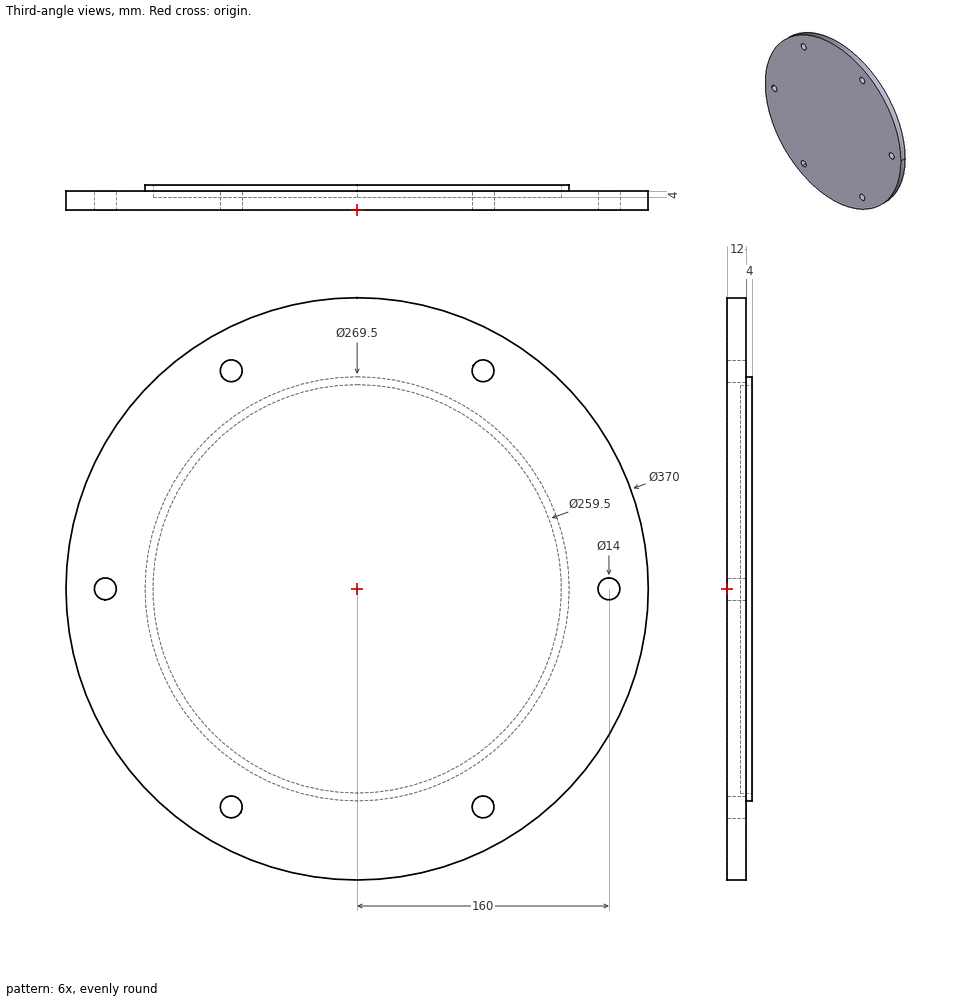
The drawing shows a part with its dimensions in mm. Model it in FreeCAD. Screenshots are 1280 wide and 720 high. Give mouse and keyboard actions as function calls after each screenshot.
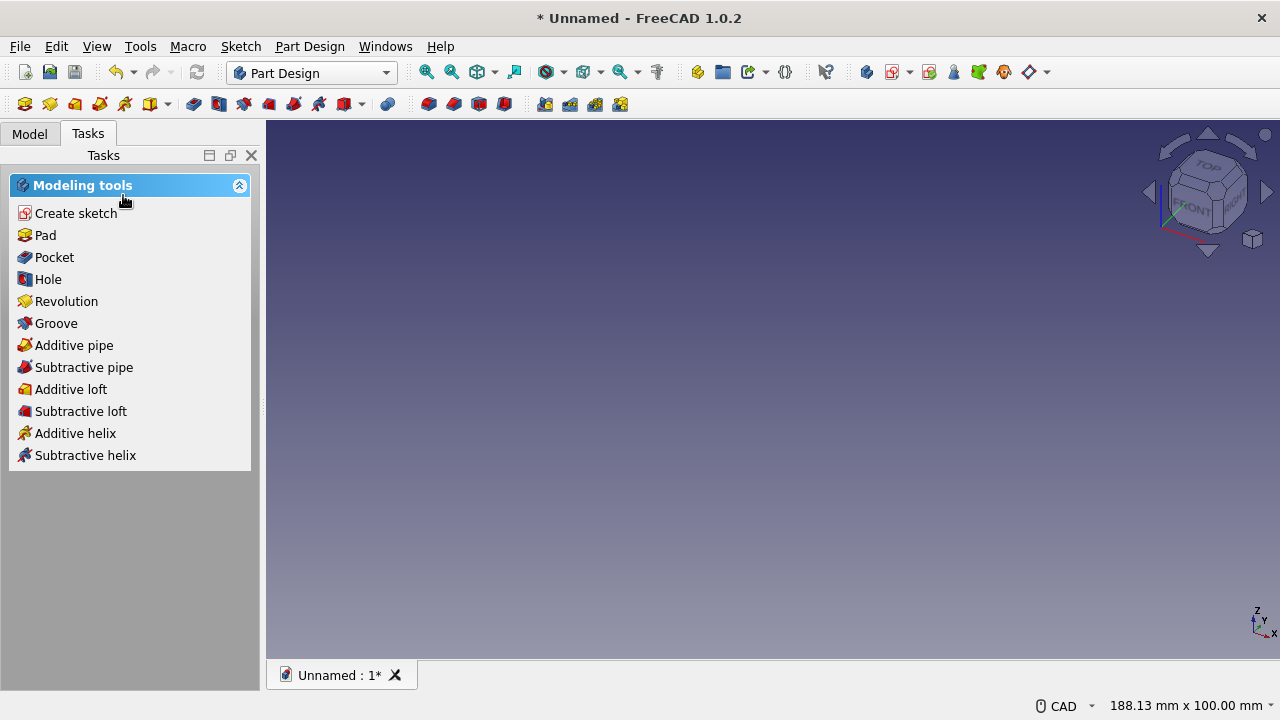
click(25, 104)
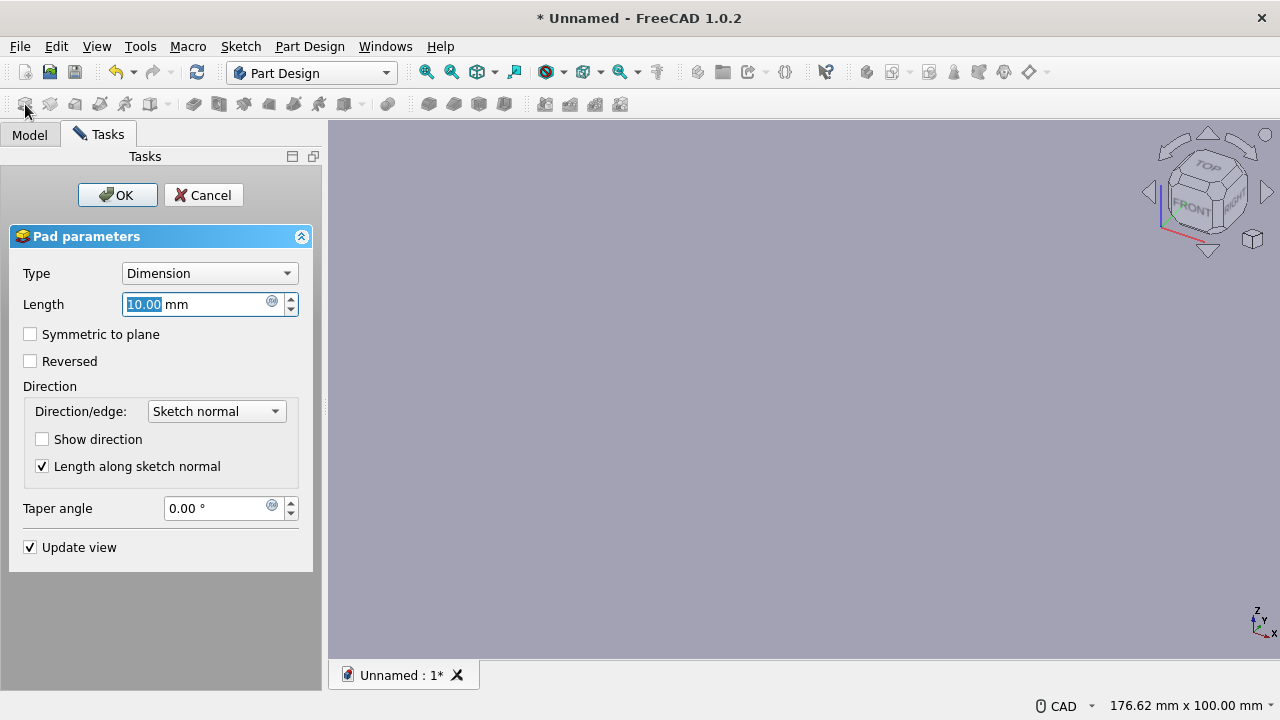
text(12)
key(Tab)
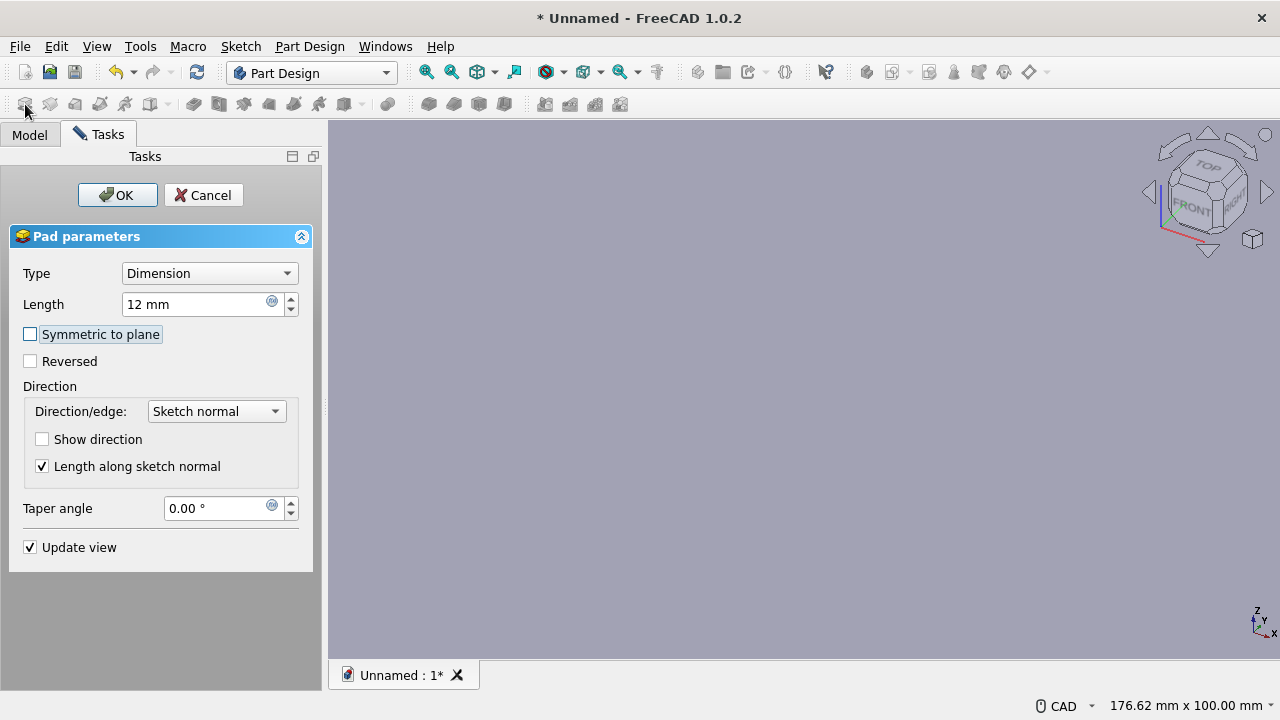
click(31, 361)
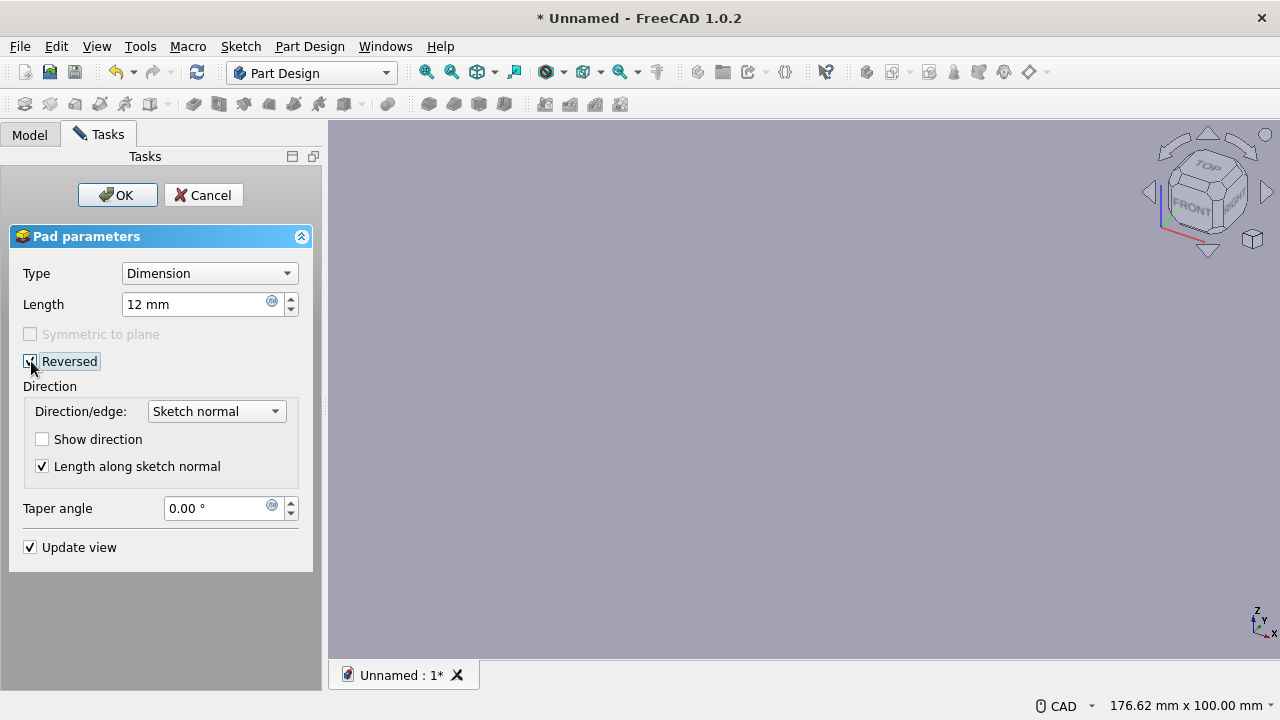
click(118, 195)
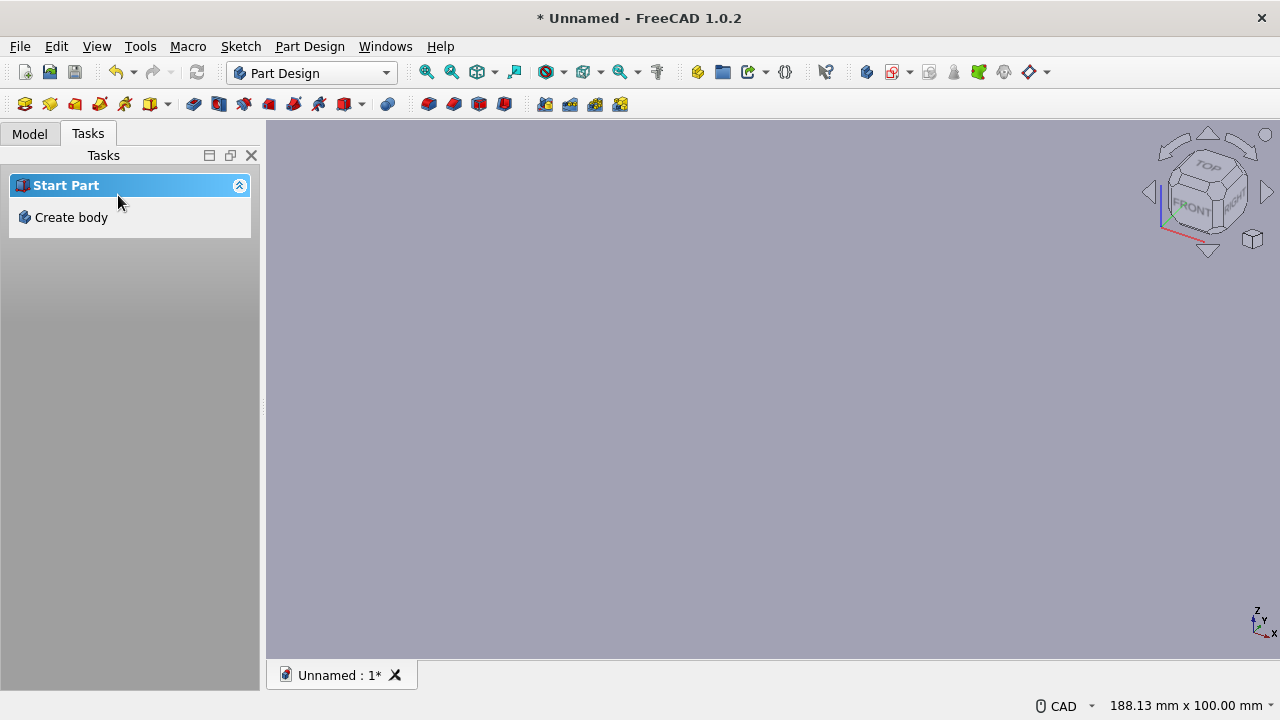
click(427, 72)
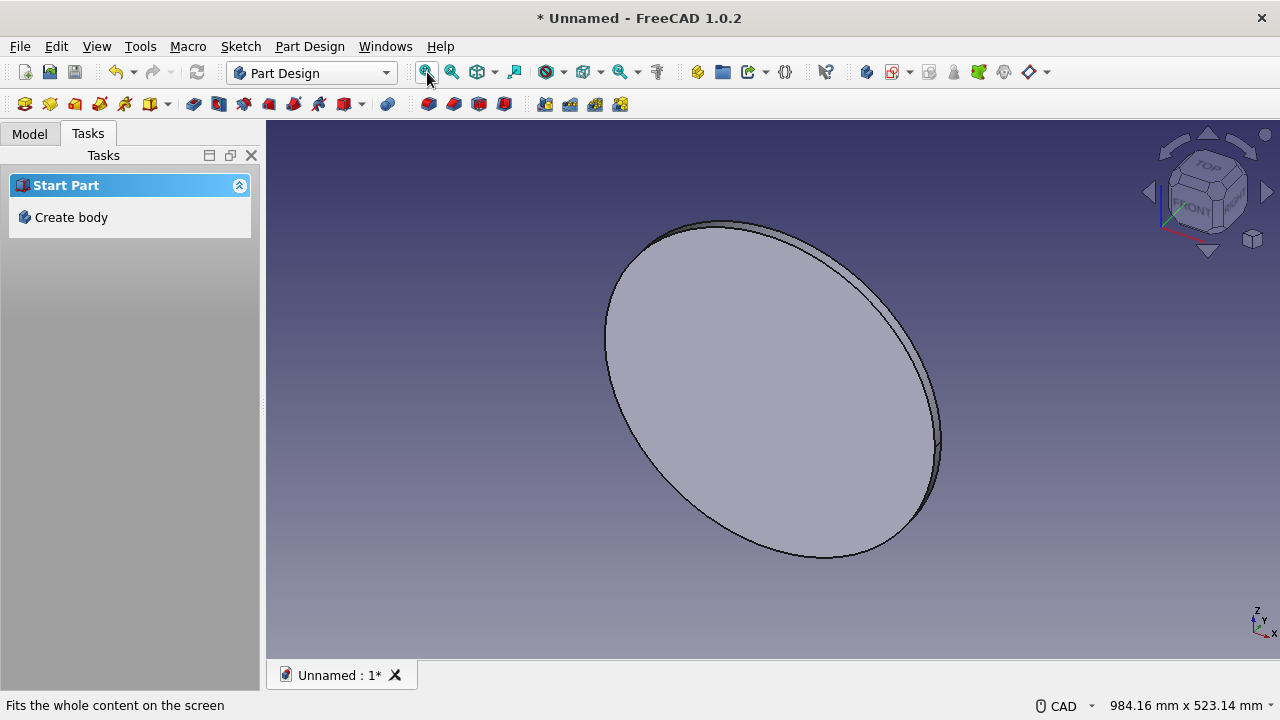
key(4)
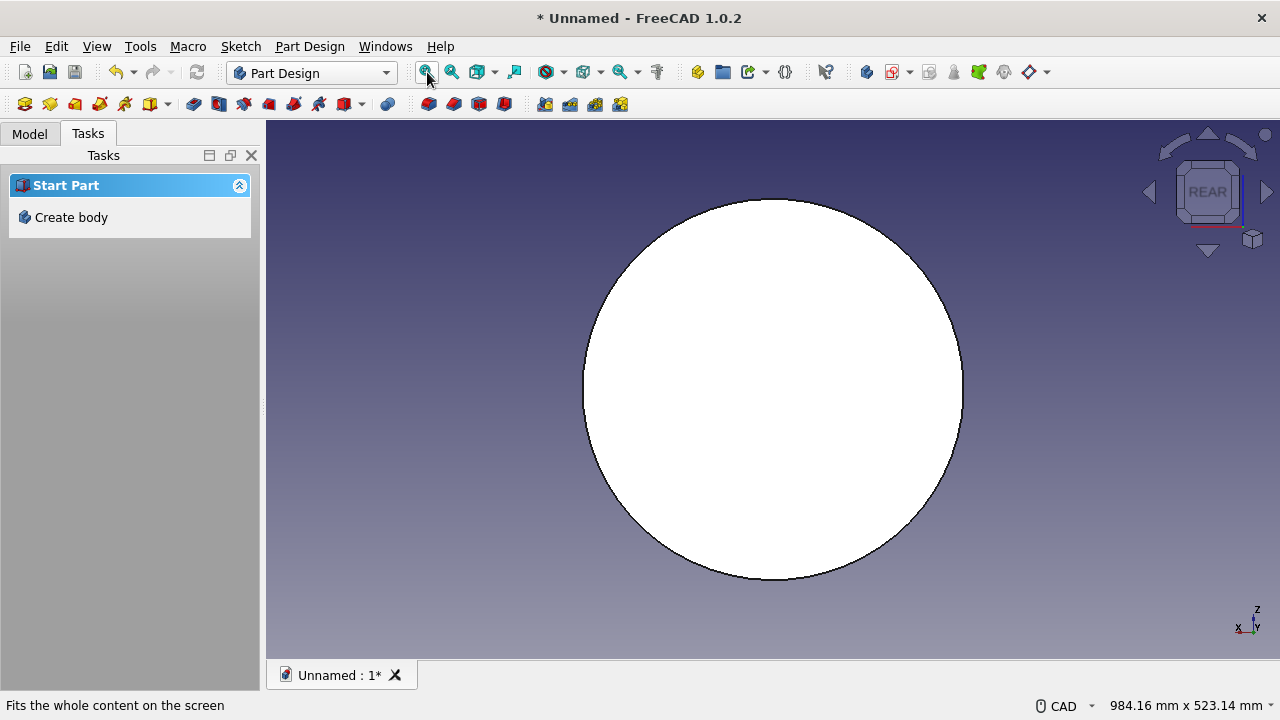
click(773, 389)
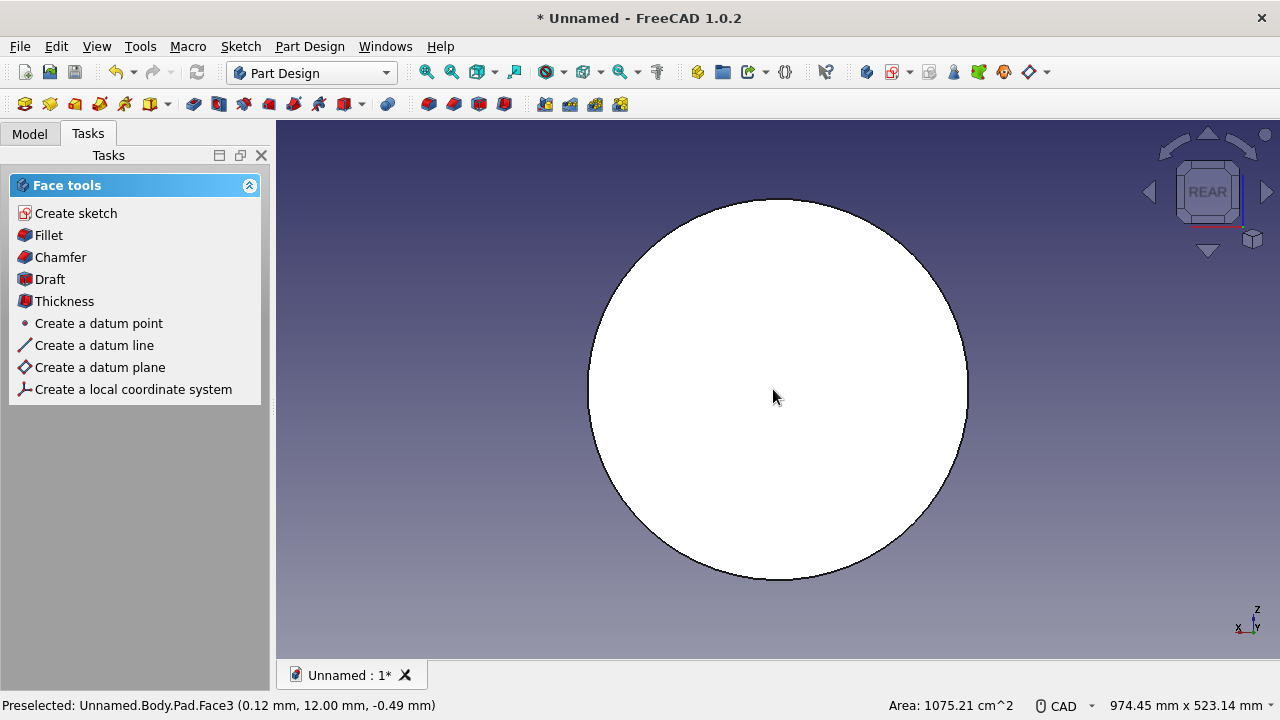
click(892, 72)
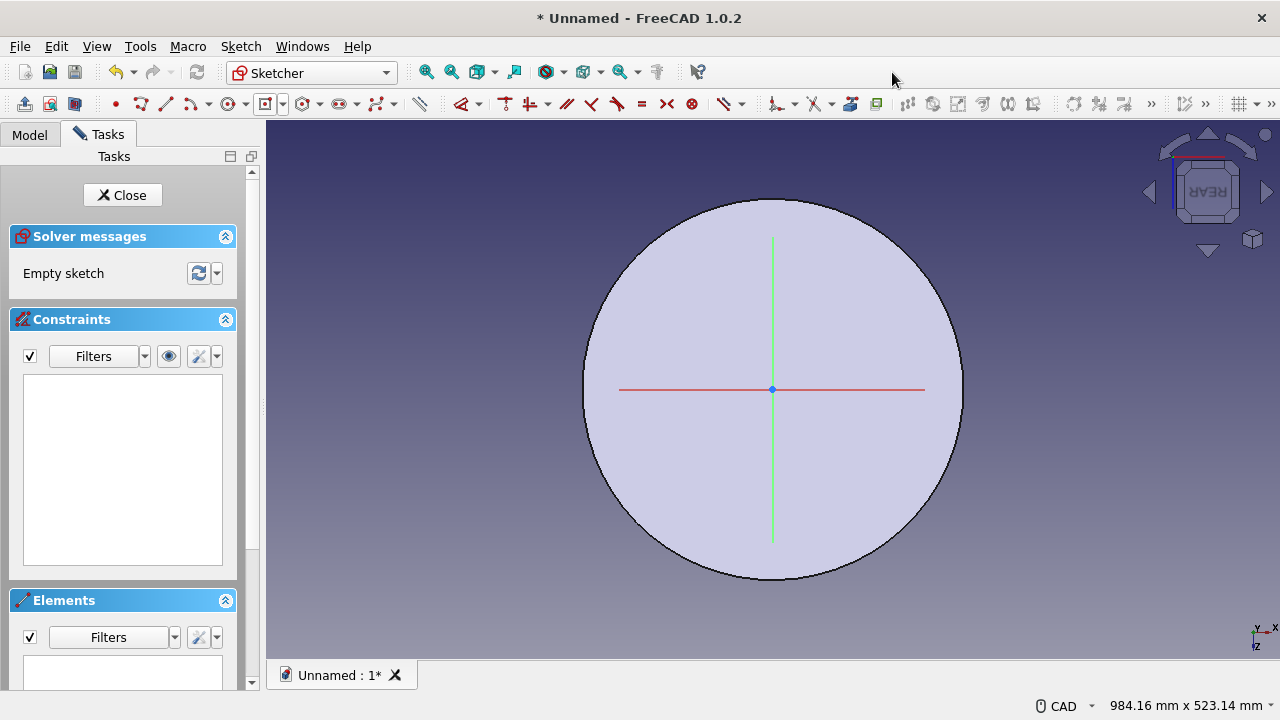
click(228, 104)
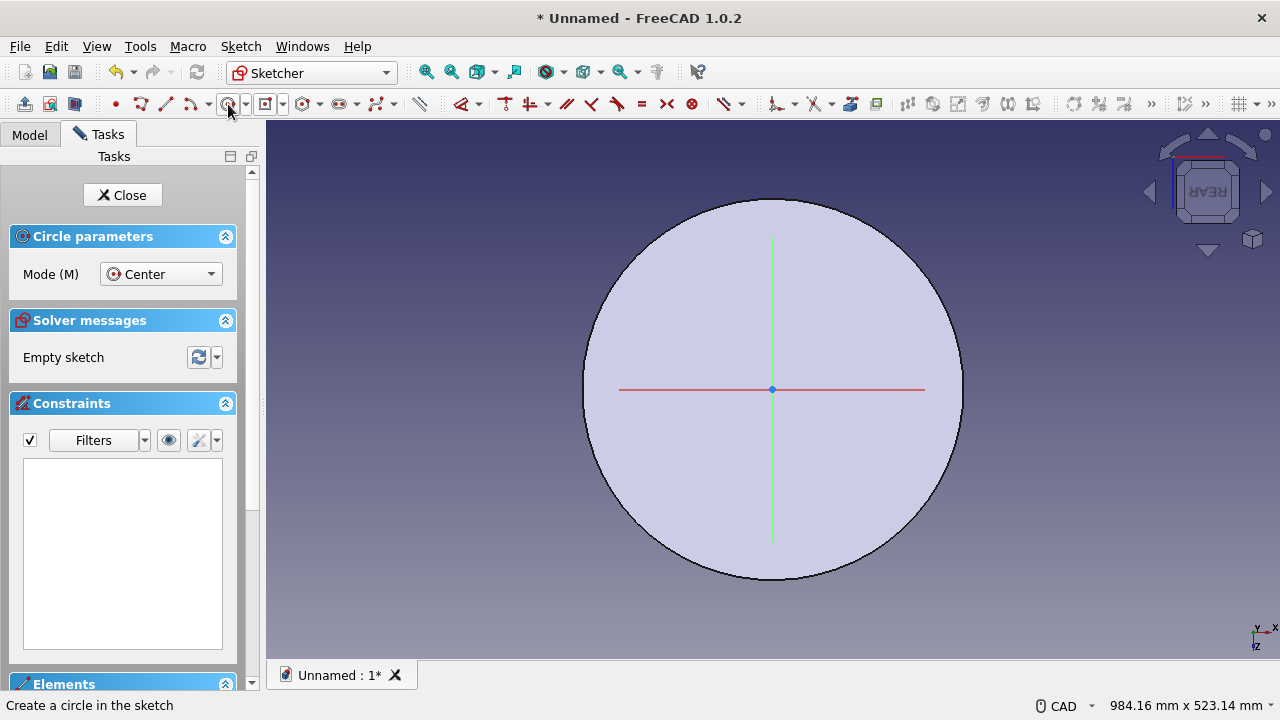
click(773, 389)
click(867, 295)
key(Escape)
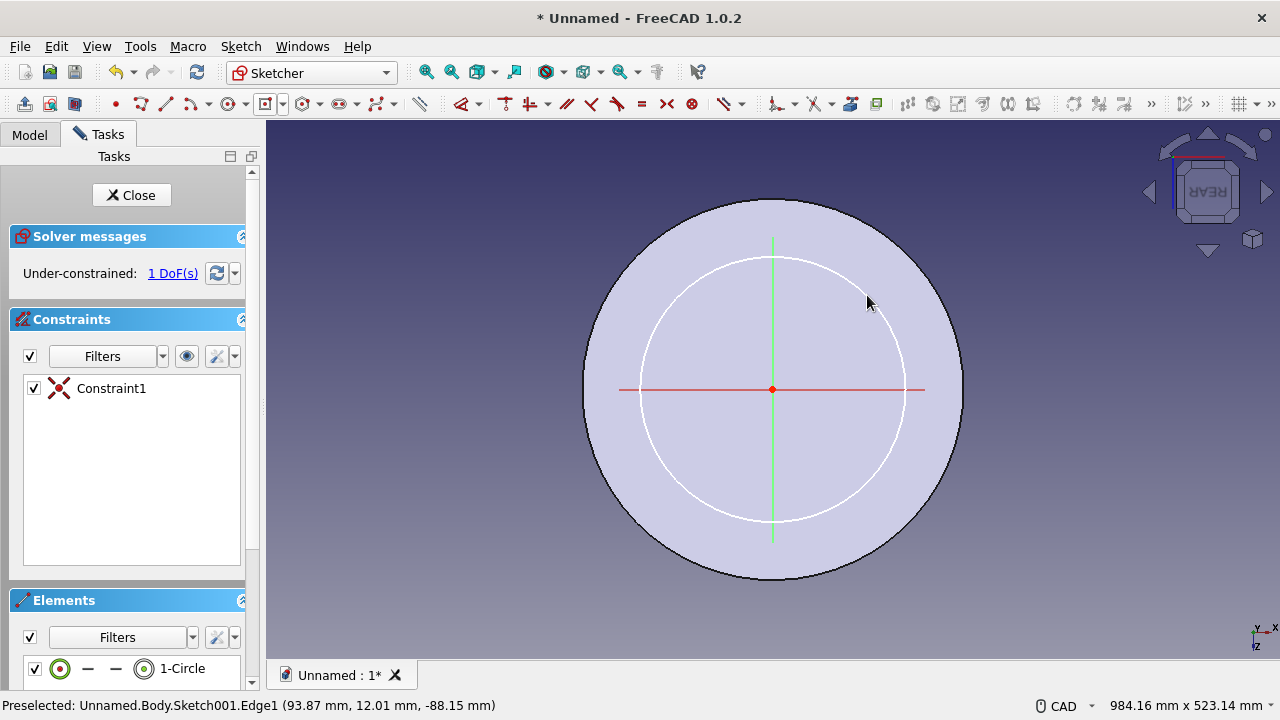
click(460, 104)